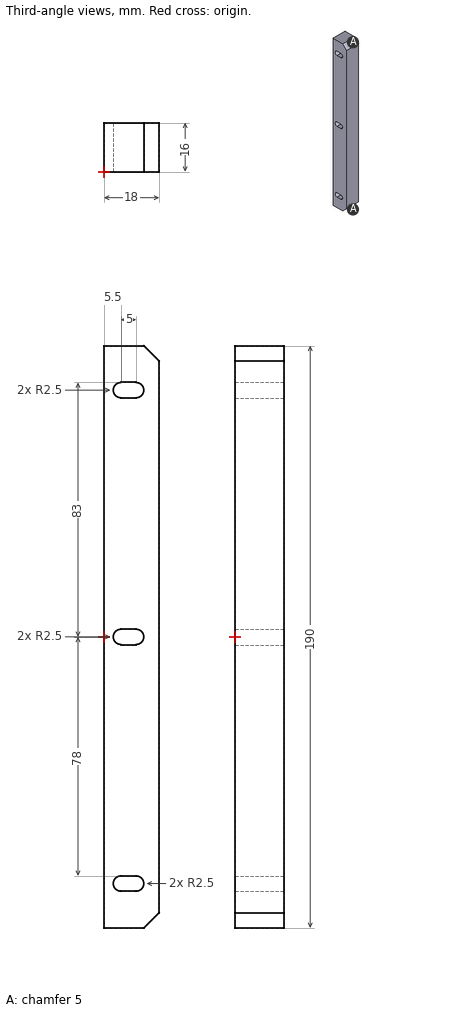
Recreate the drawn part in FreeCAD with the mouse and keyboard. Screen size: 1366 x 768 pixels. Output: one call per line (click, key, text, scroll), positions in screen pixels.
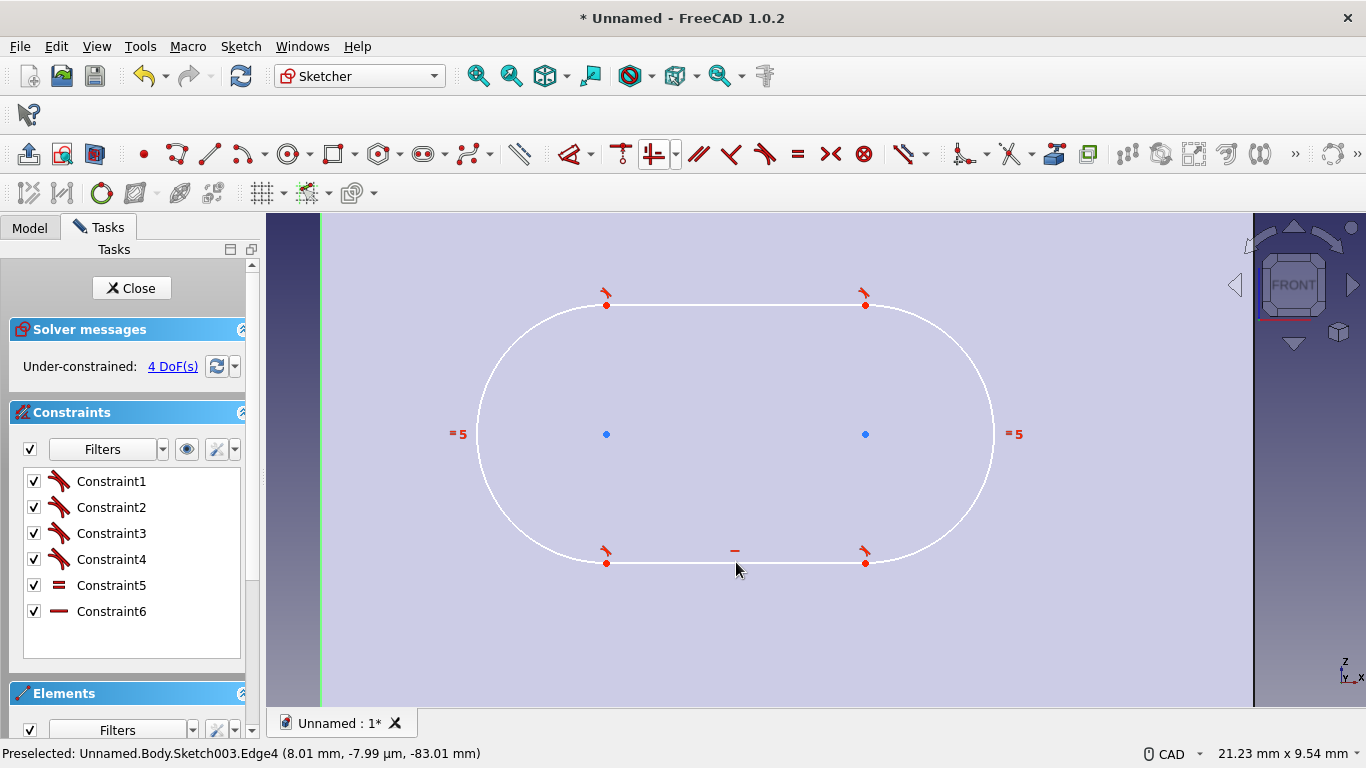
click(568, 154)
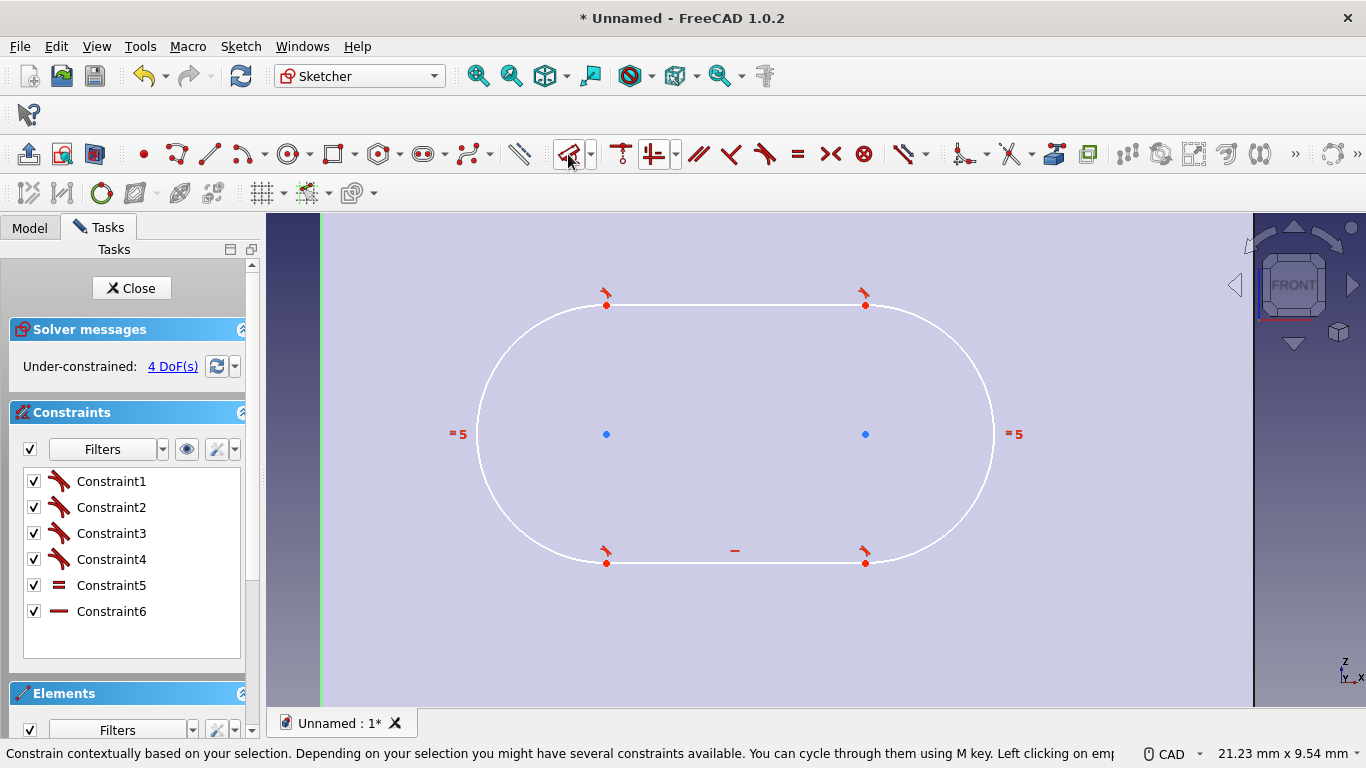
click(502, 358)
click(476, 339)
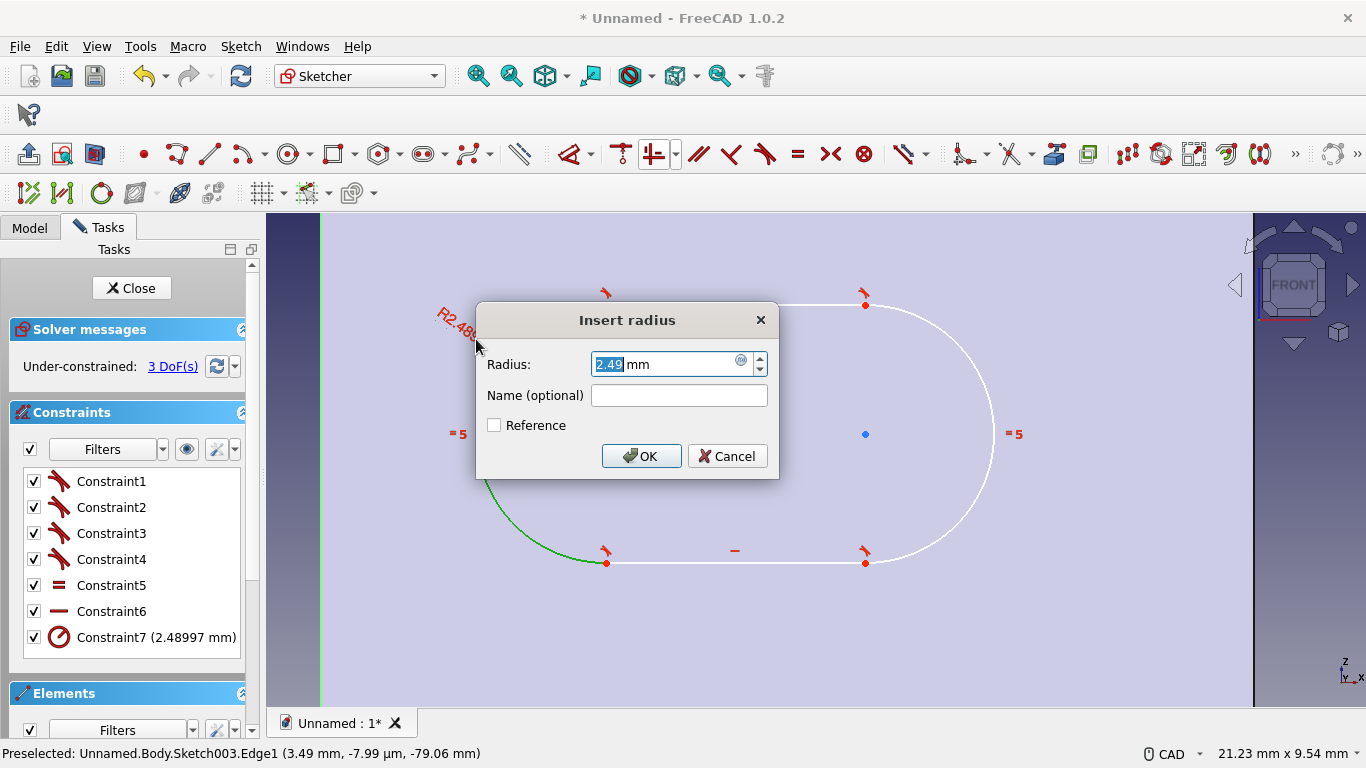
text(2.5)
key(Return)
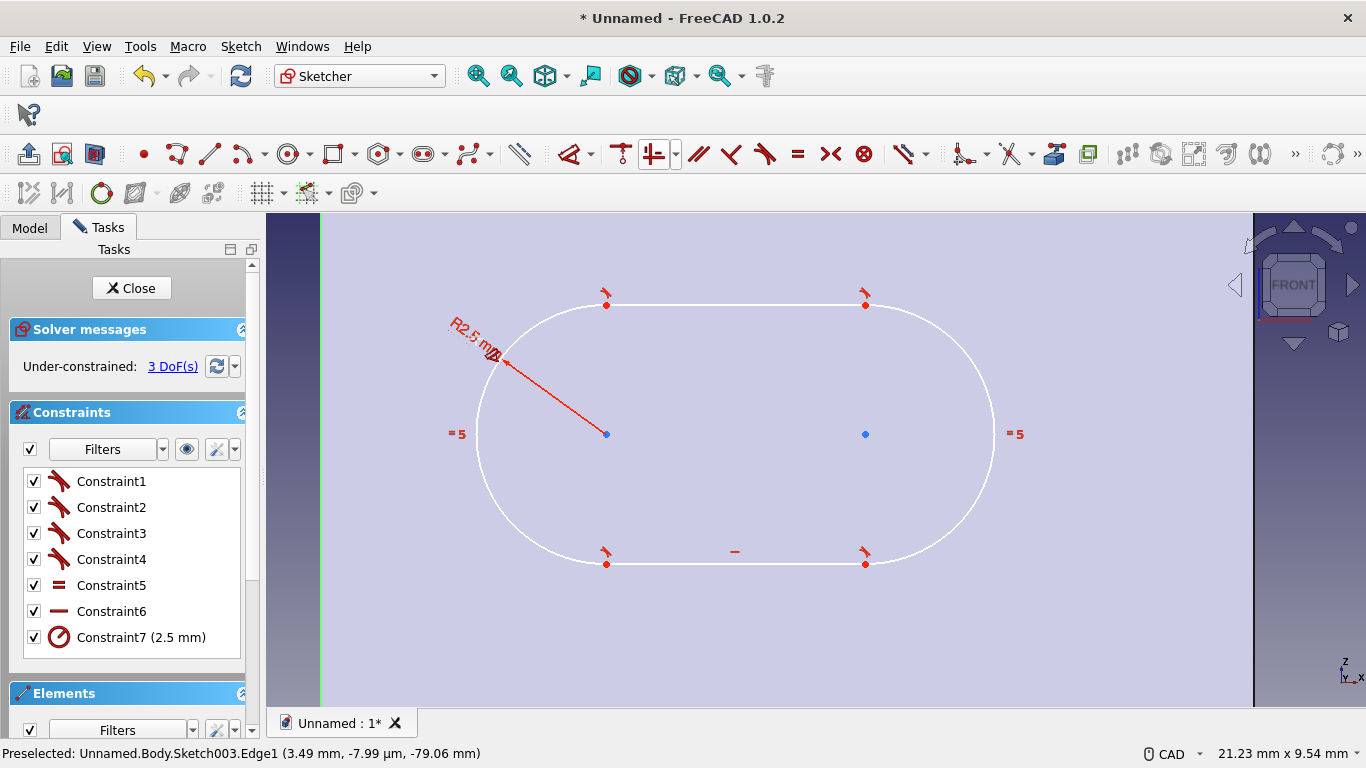
click(684, 305)
click(736, 271)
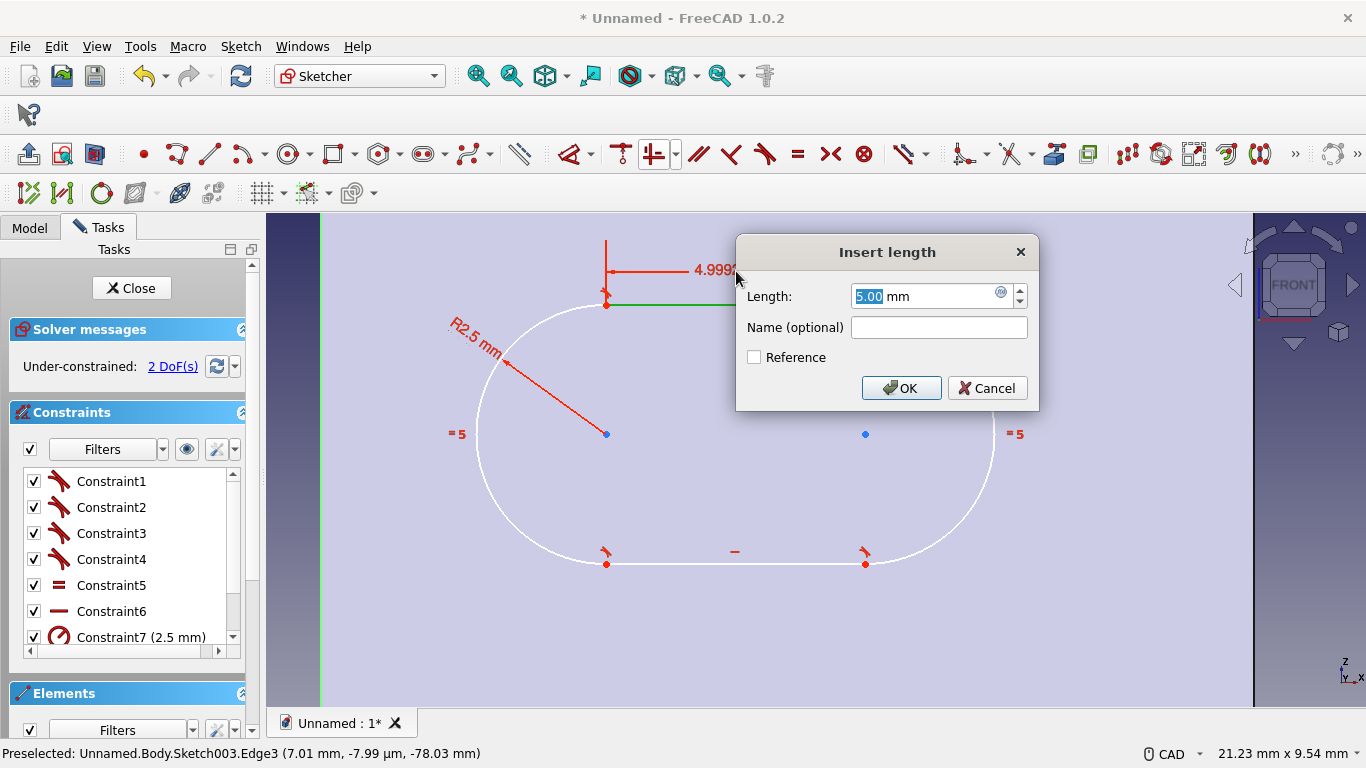
text(5)
key(Return)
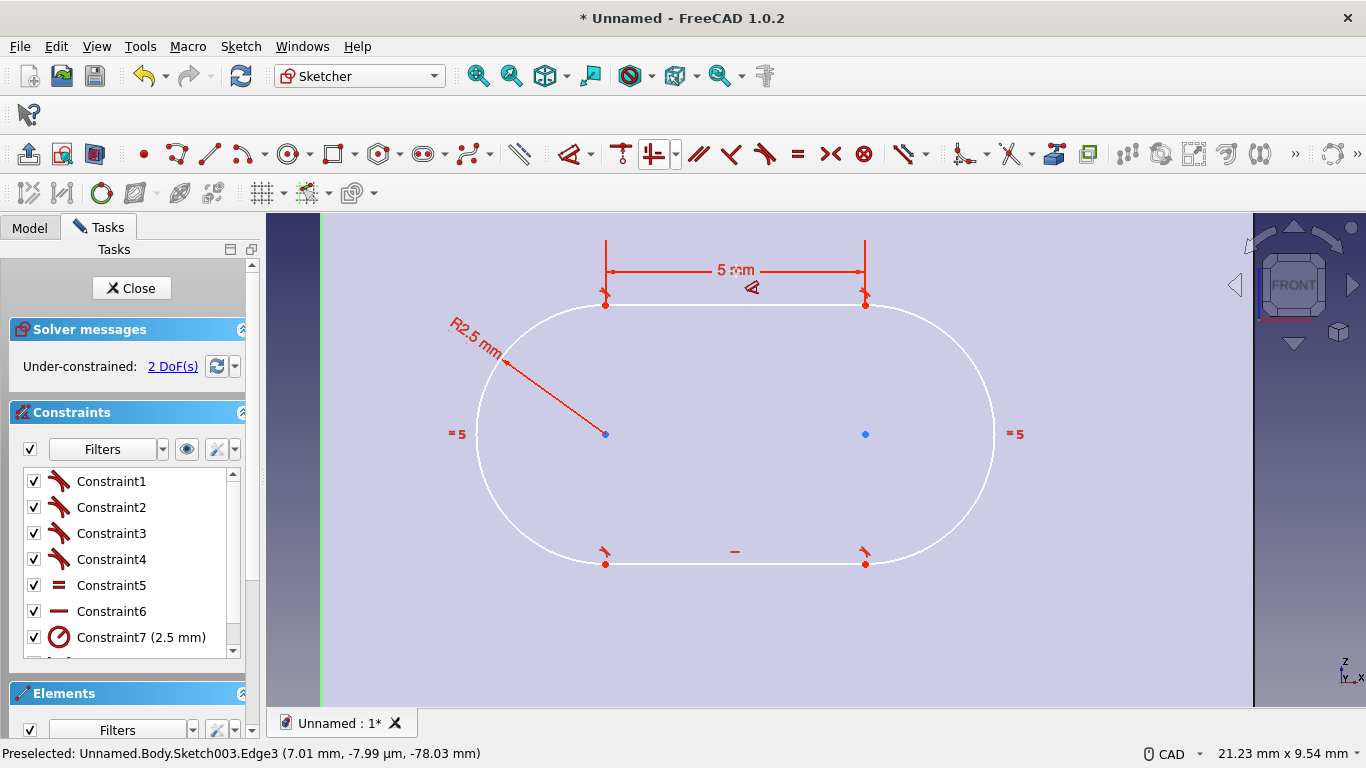
click(606, 305)
click(640, 273)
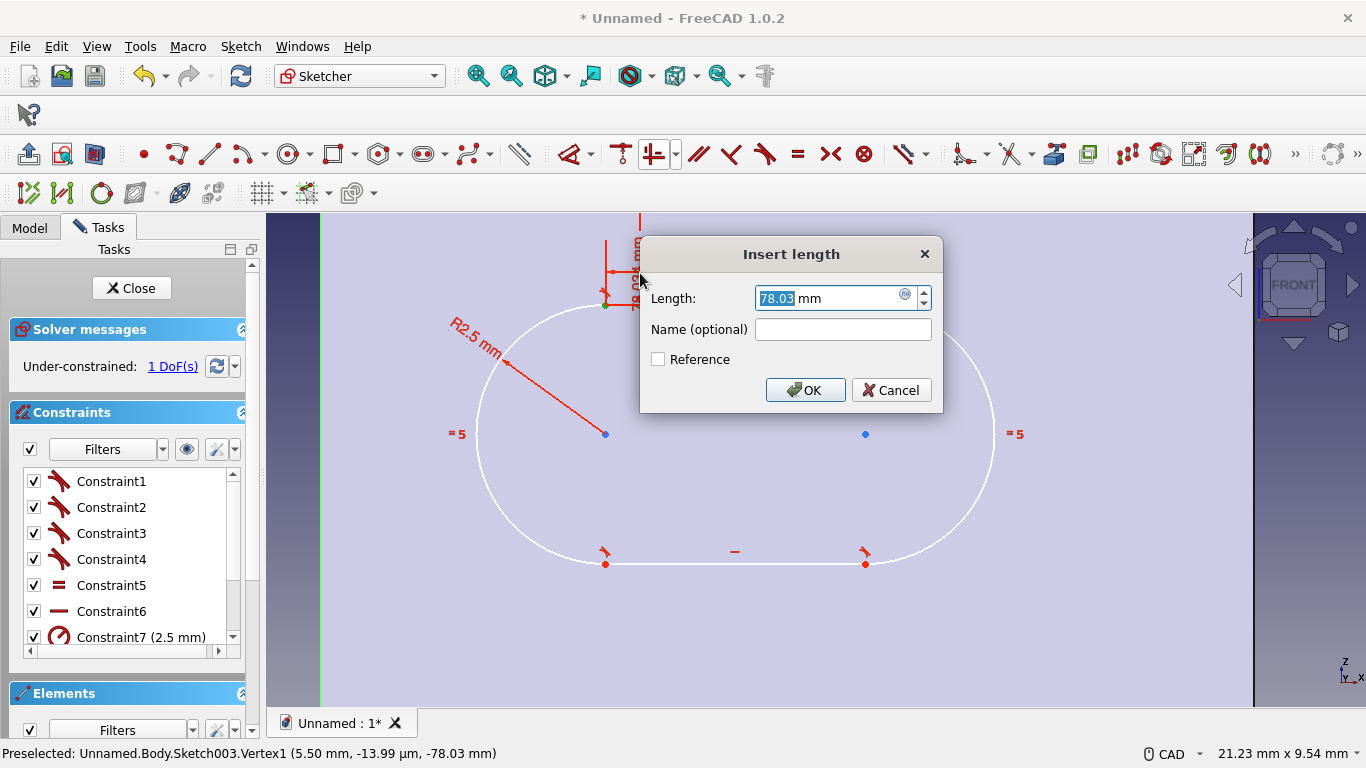
text(78)
key(Return)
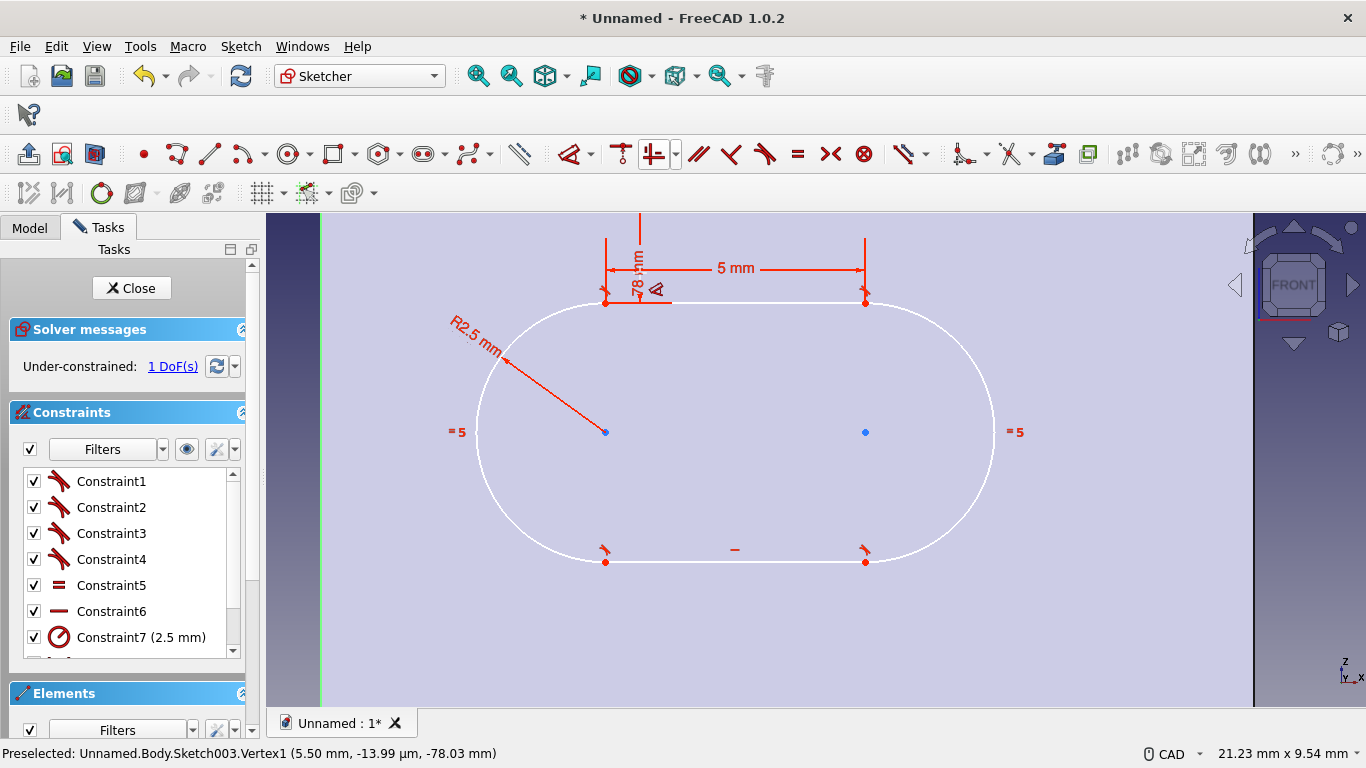
click(606, 303)
click(398, 337)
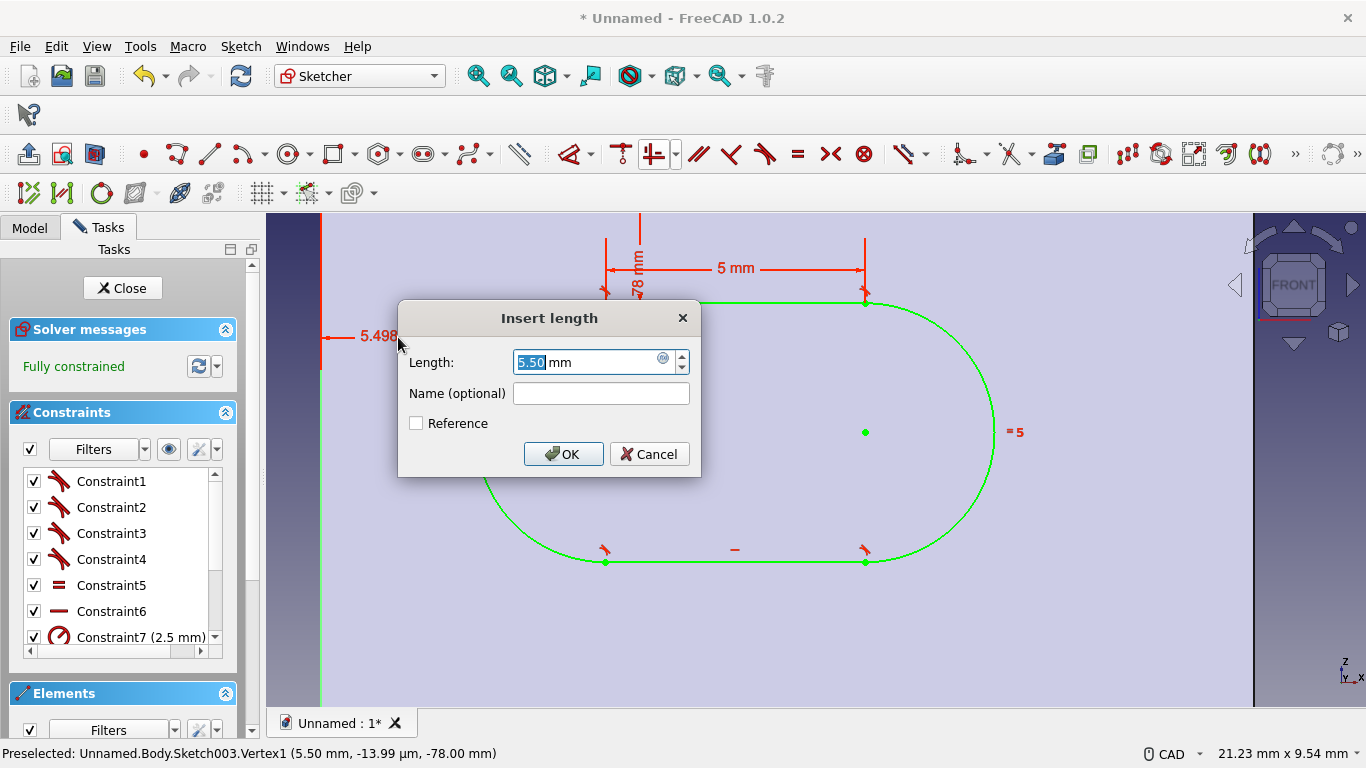
text(5.5)
key(Return)
key(Escape)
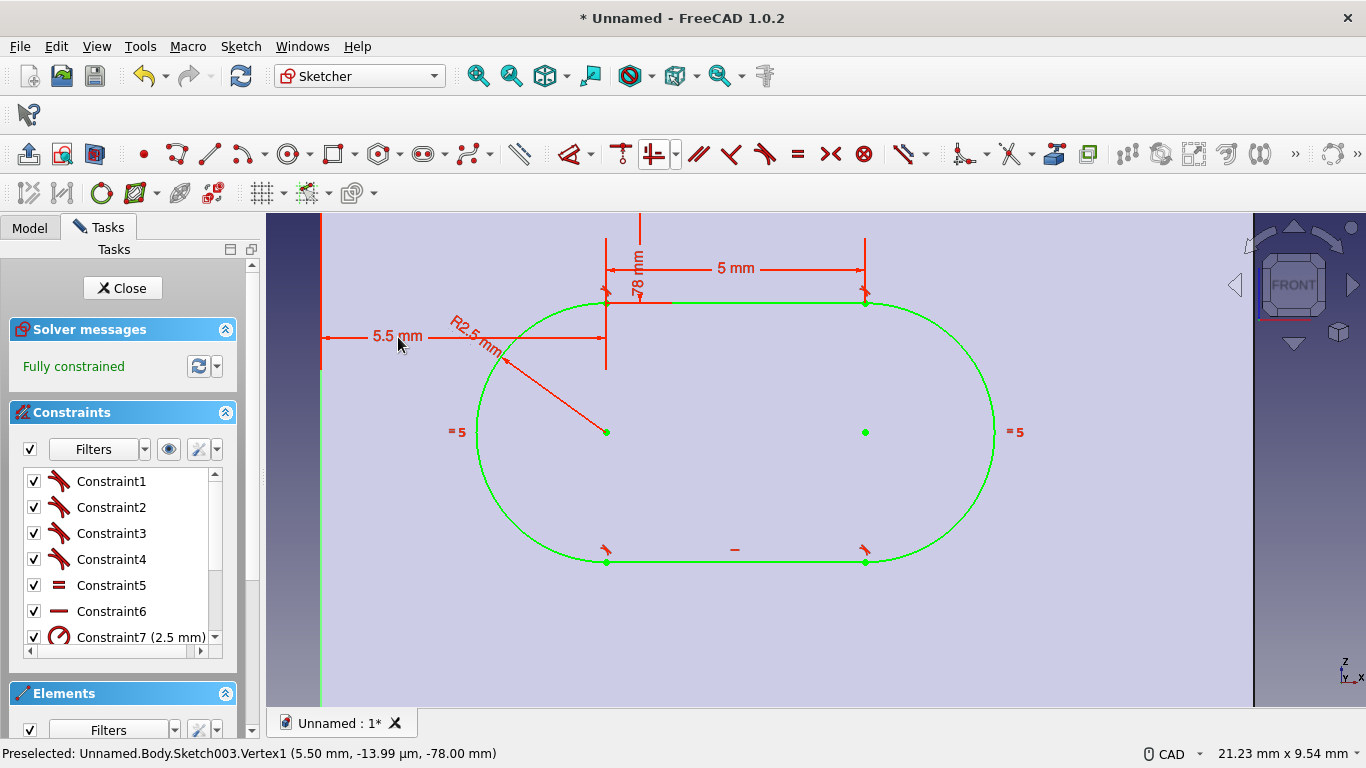
click(123, 288)